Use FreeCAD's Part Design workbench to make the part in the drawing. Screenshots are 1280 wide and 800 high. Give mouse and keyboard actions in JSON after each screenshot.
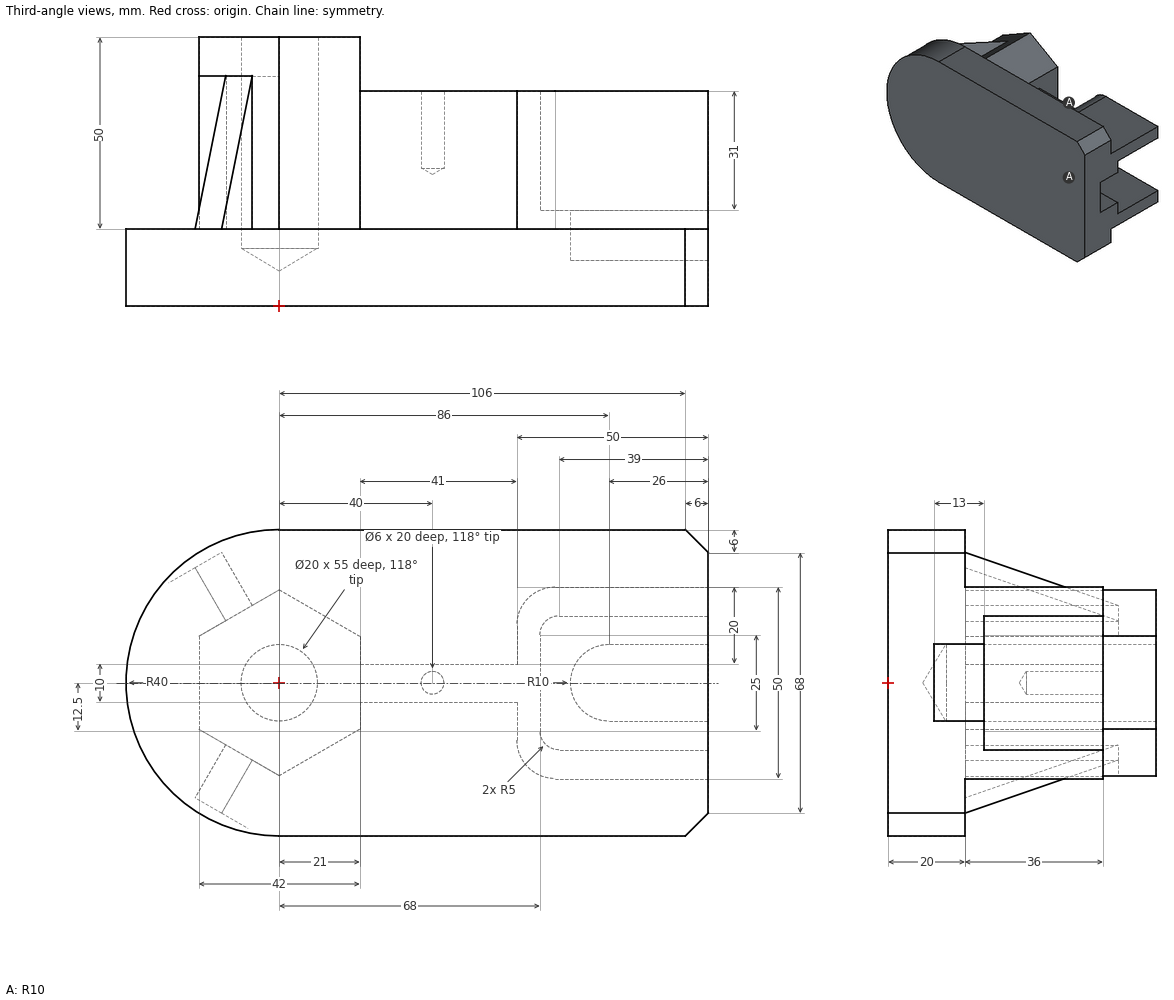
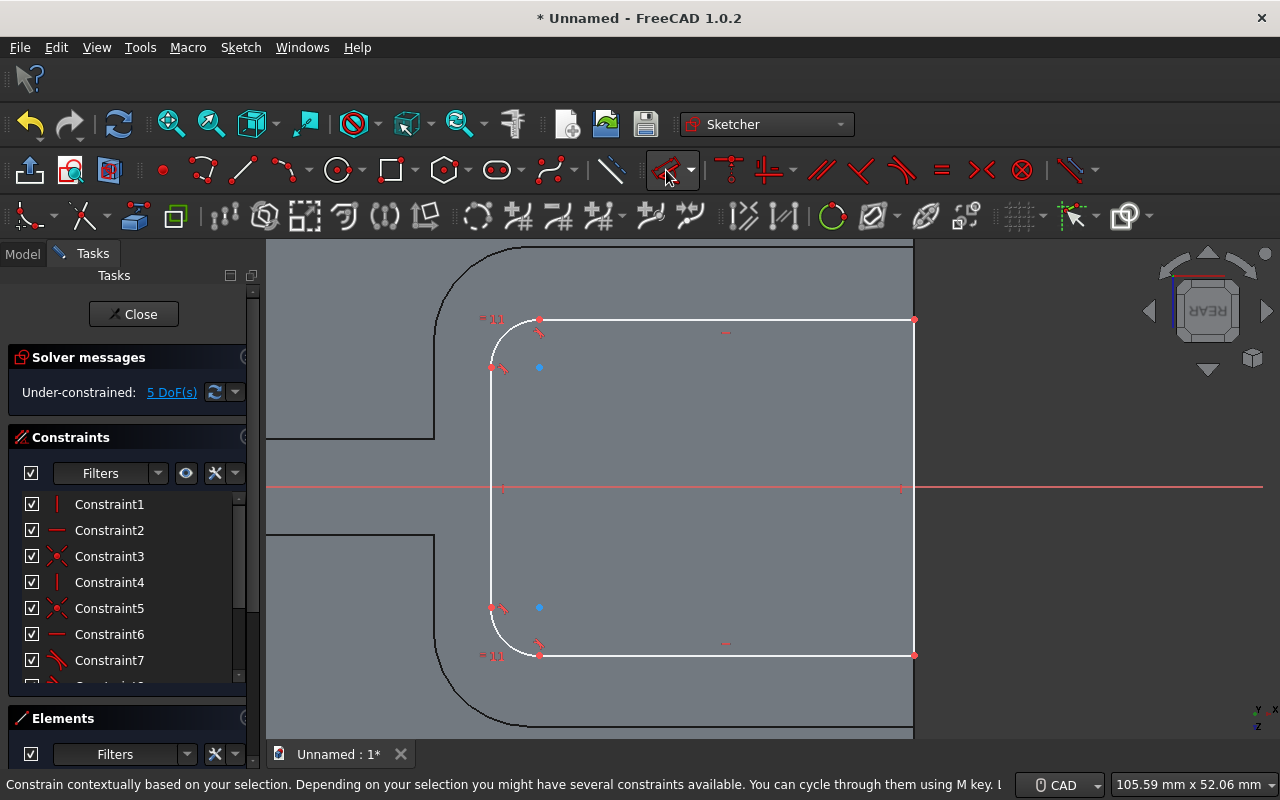
{"action": "left_click", "coordinate": [496, 630]}
{"action": "left_click", "coordinate": [468, 645]}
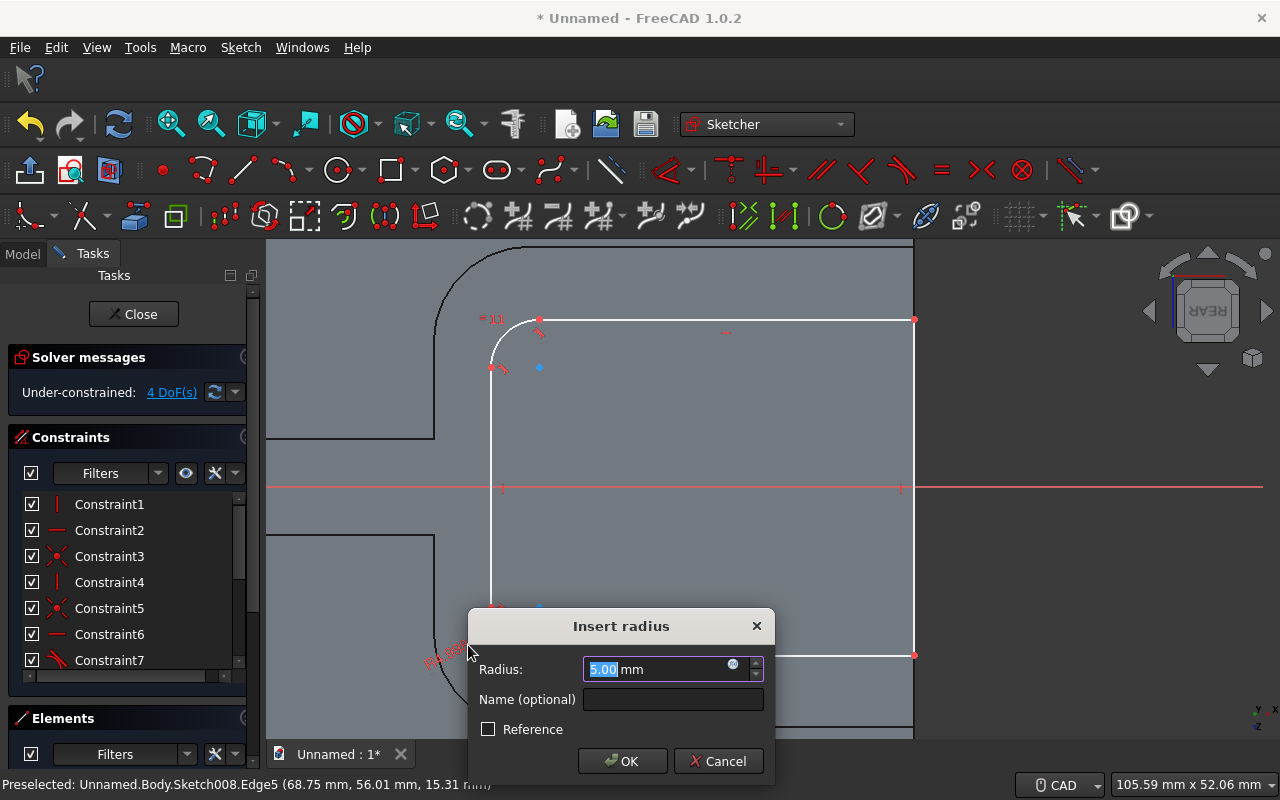
{"action": "type", "text": "5"}
{"action": "key", "text": "Return"}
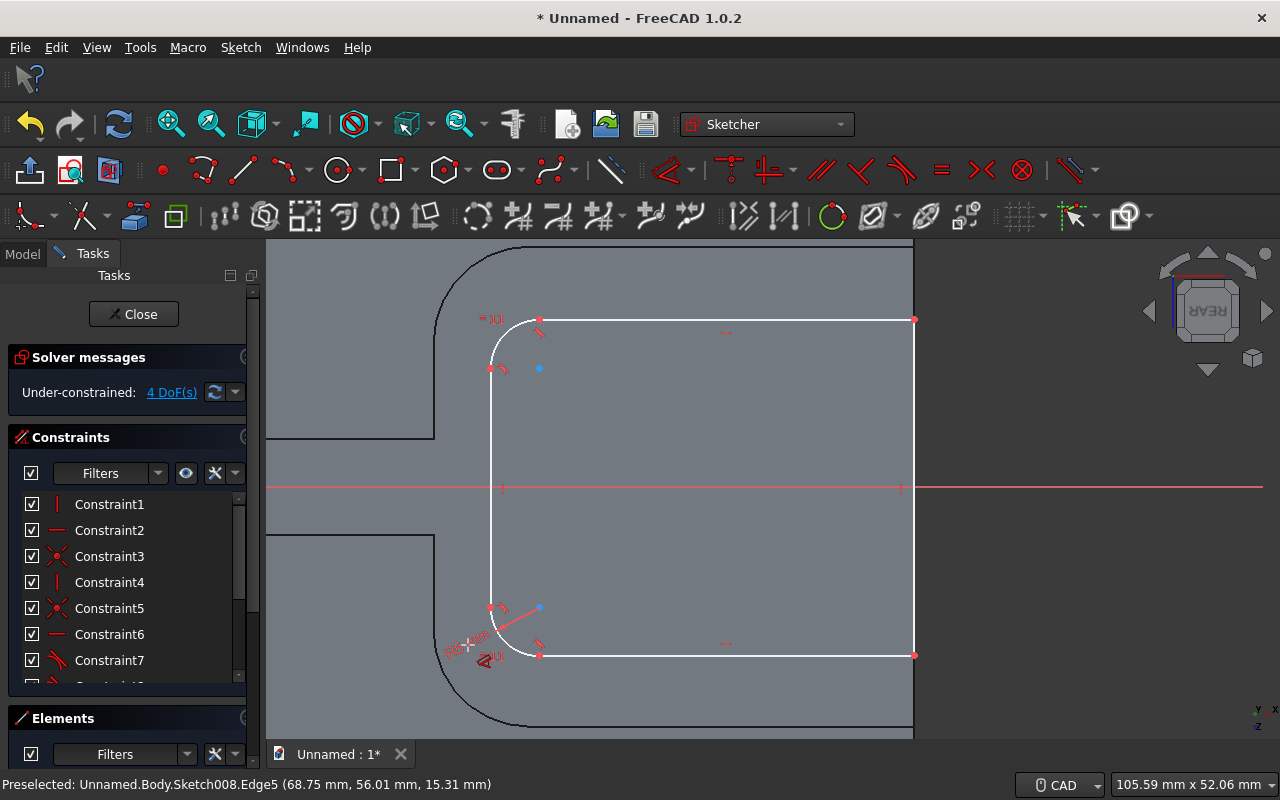
{"action": "left_click", "coordinate": [491, 440]}
{"action": "left_click", "coordinate": [457, 433]}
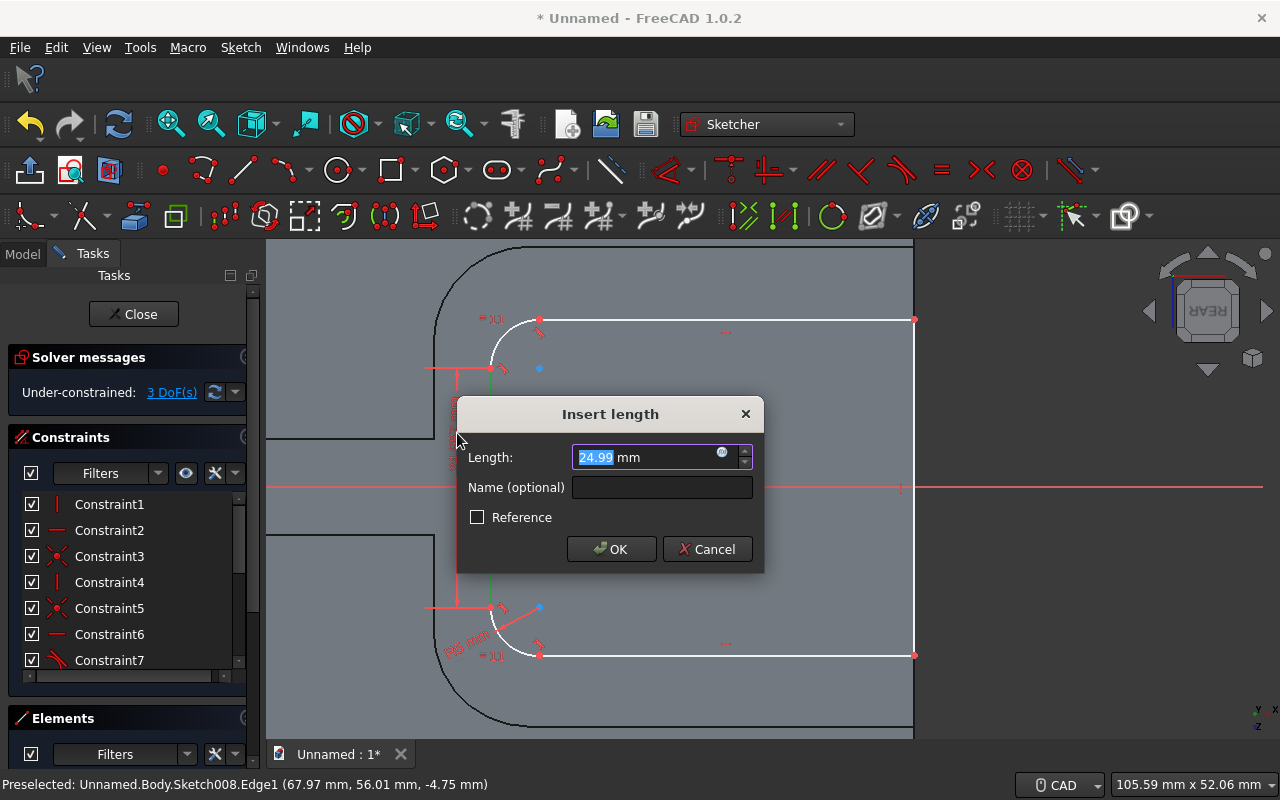
{"action": "type", "text": "25"}
{"action": "key", "text": "Return"}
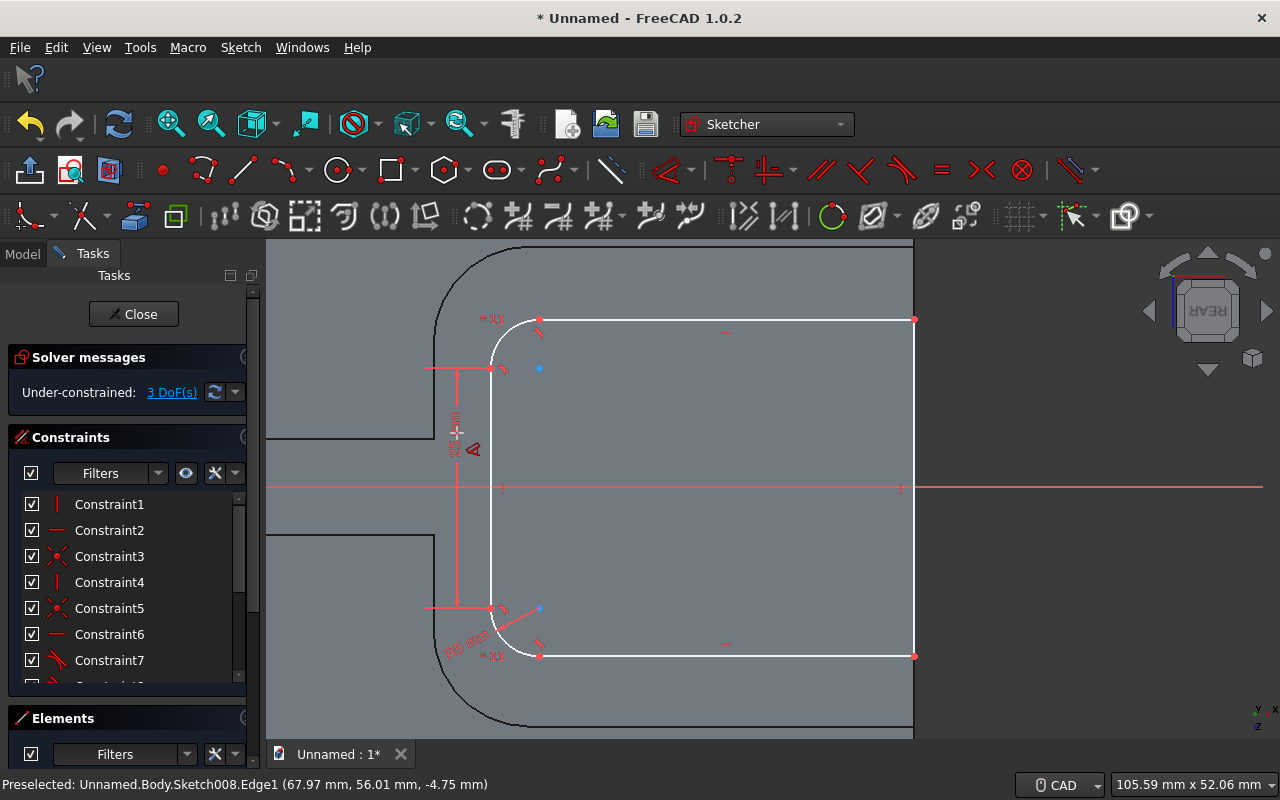
{"action": "left_click", "coordinate": [652, 656]}
{"action": "left_click", "coordinate": [726, 690]}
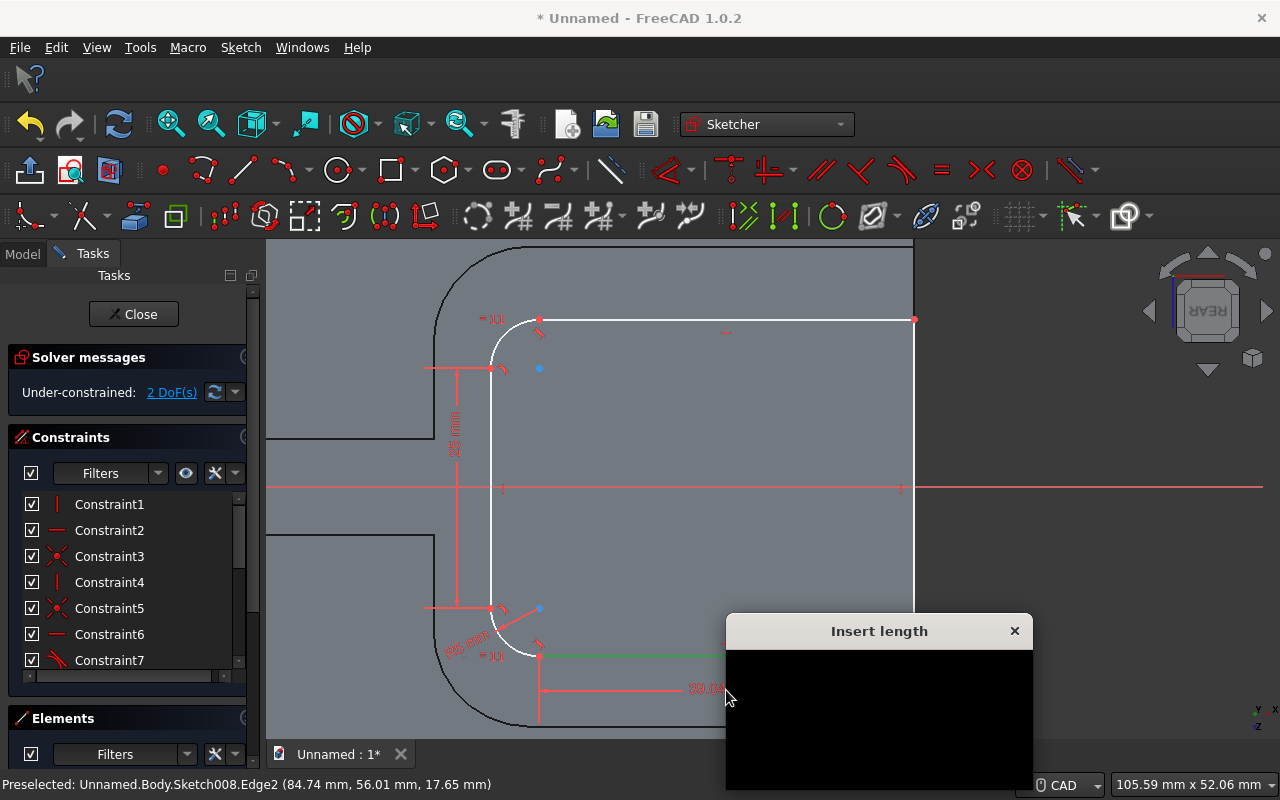
{"action": "type", "text": "39"}
{"action": "key", "text": "Return"}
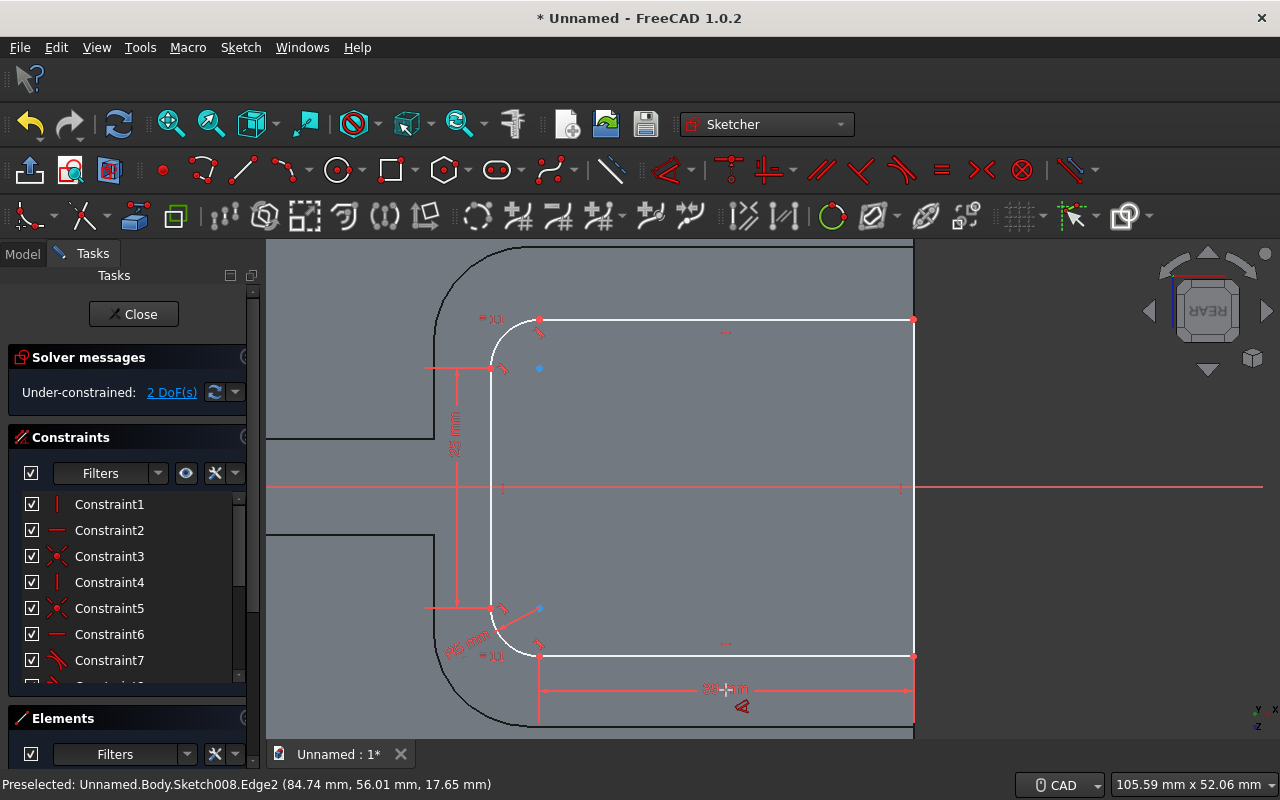
{"action": "left_click", "coordinate": [491, 368]}
{"action": "left_click", "coordinate": [392, 334]}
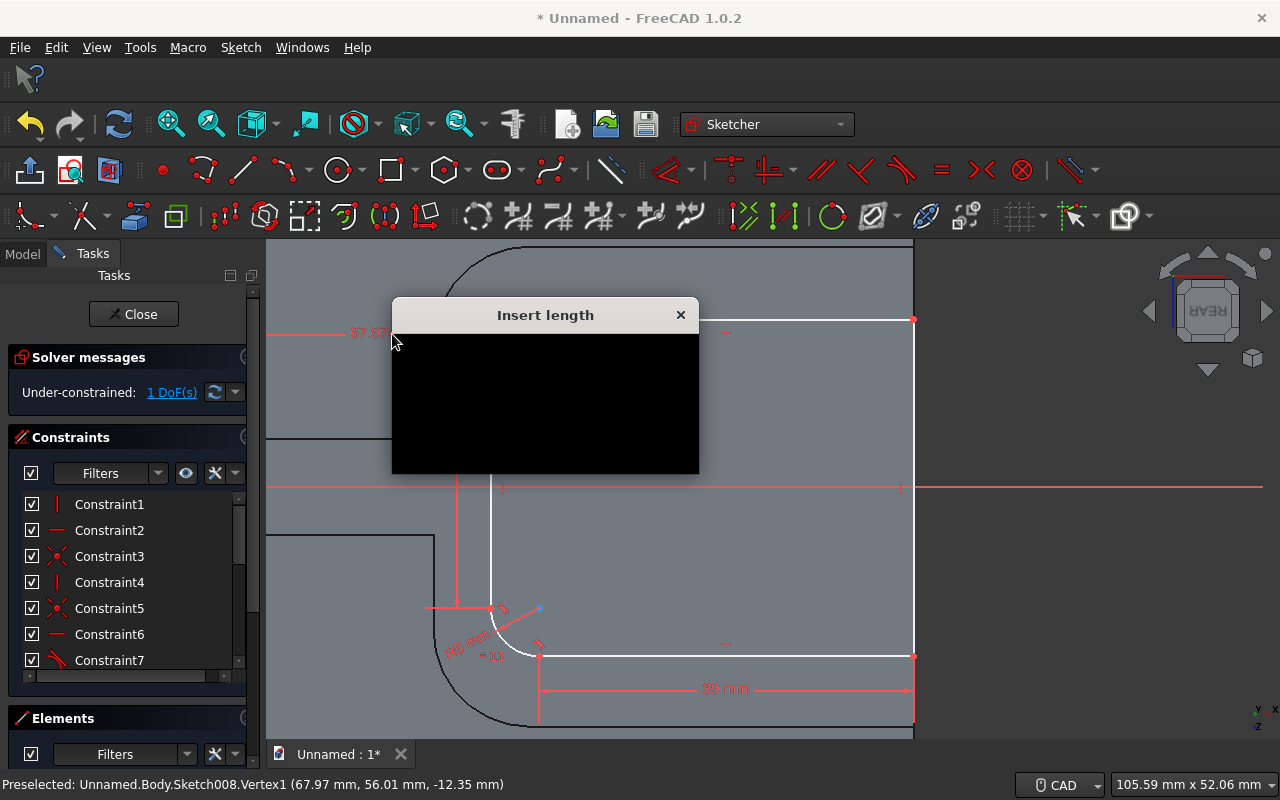
{"action": "type", "text": "68"}
{"action": "key", "text": "Return"}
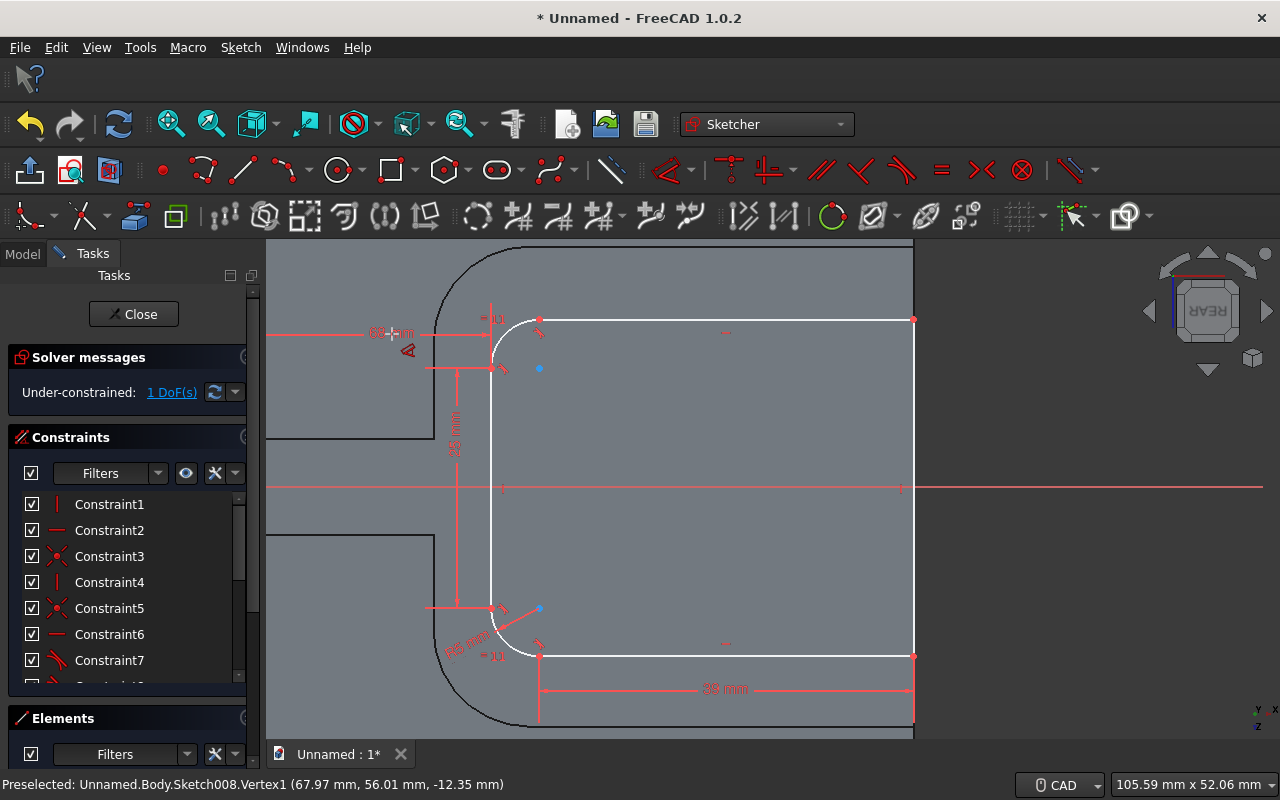
{"action": "left_click", "coordinate": [491, 368]}
{"action": "left_click", "coordinate": [525, 400]}